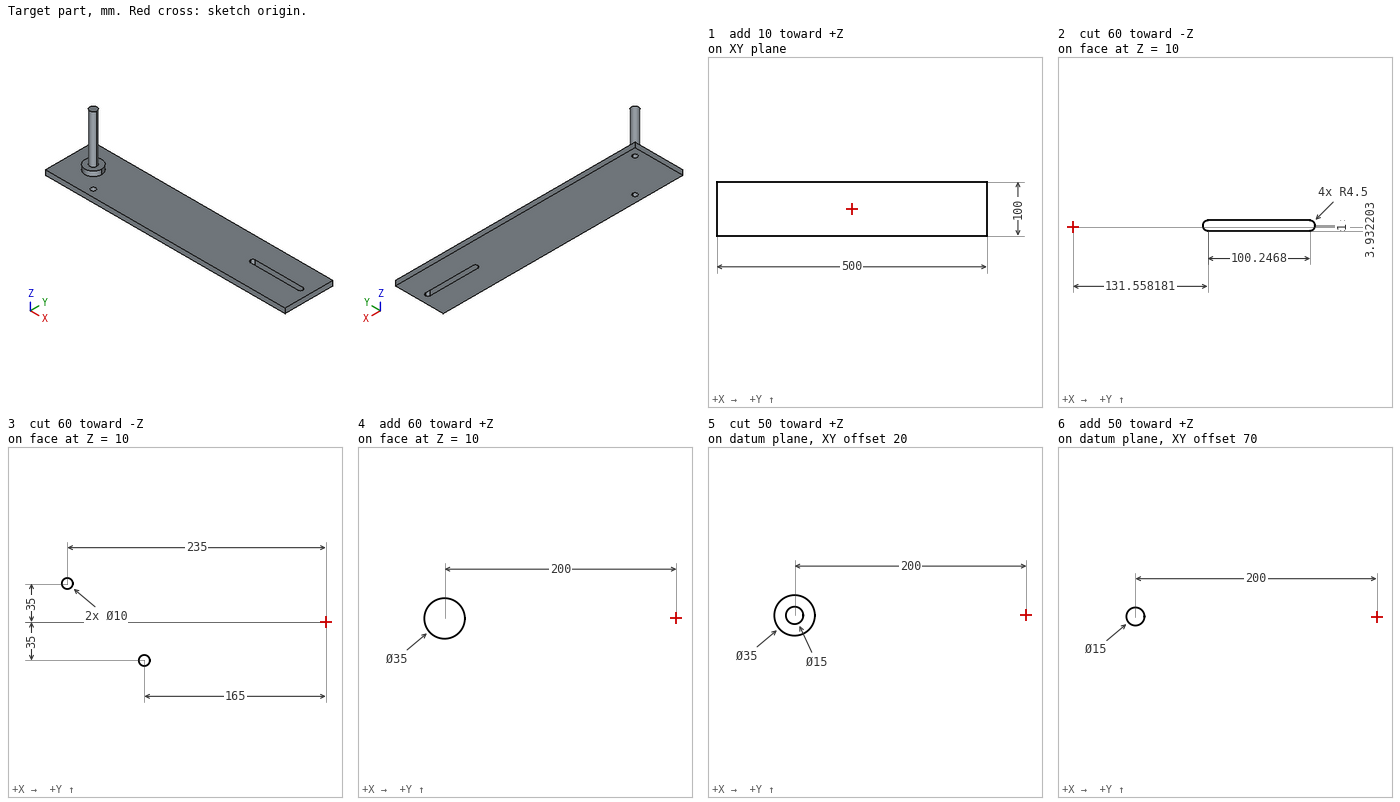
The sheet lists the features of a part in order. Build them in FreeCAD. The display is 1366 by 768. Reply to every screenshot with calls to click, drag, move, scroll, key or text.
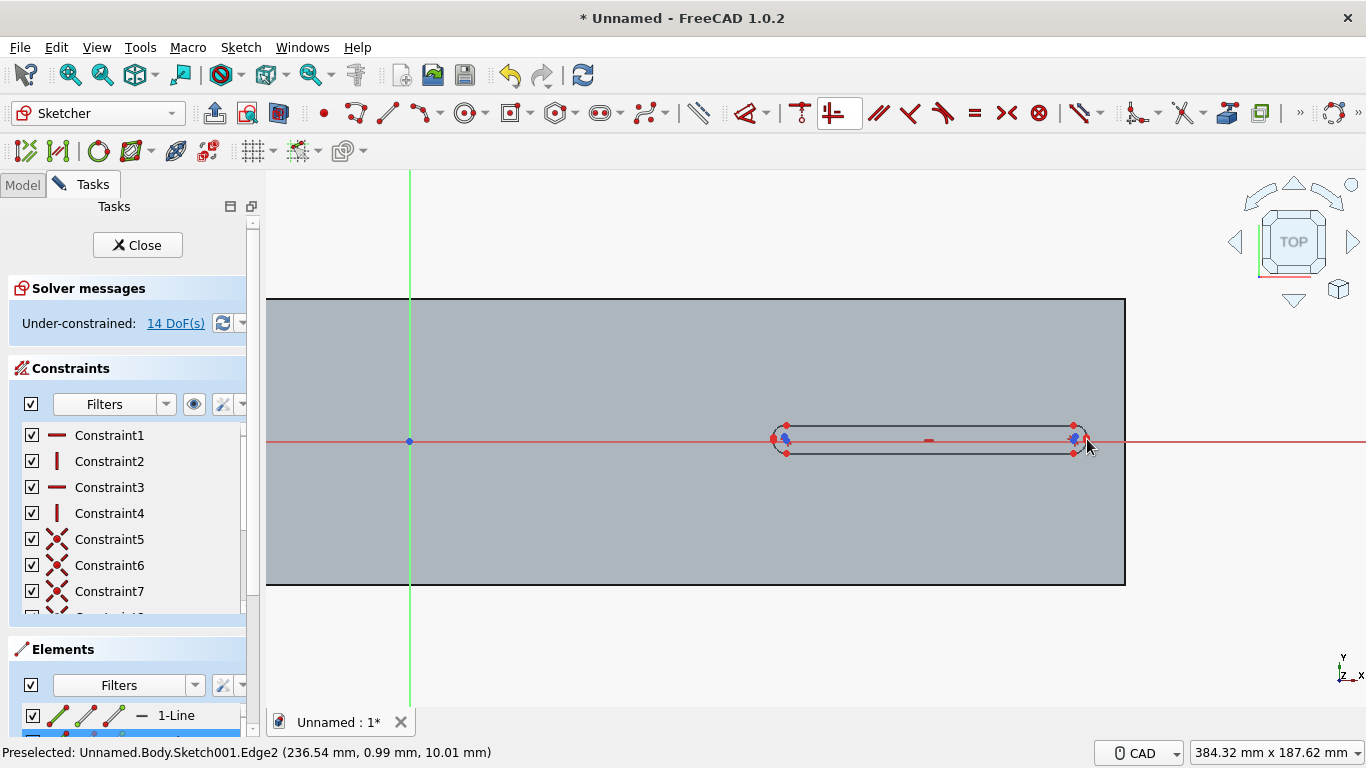
scroll(1079, 452, up, 5)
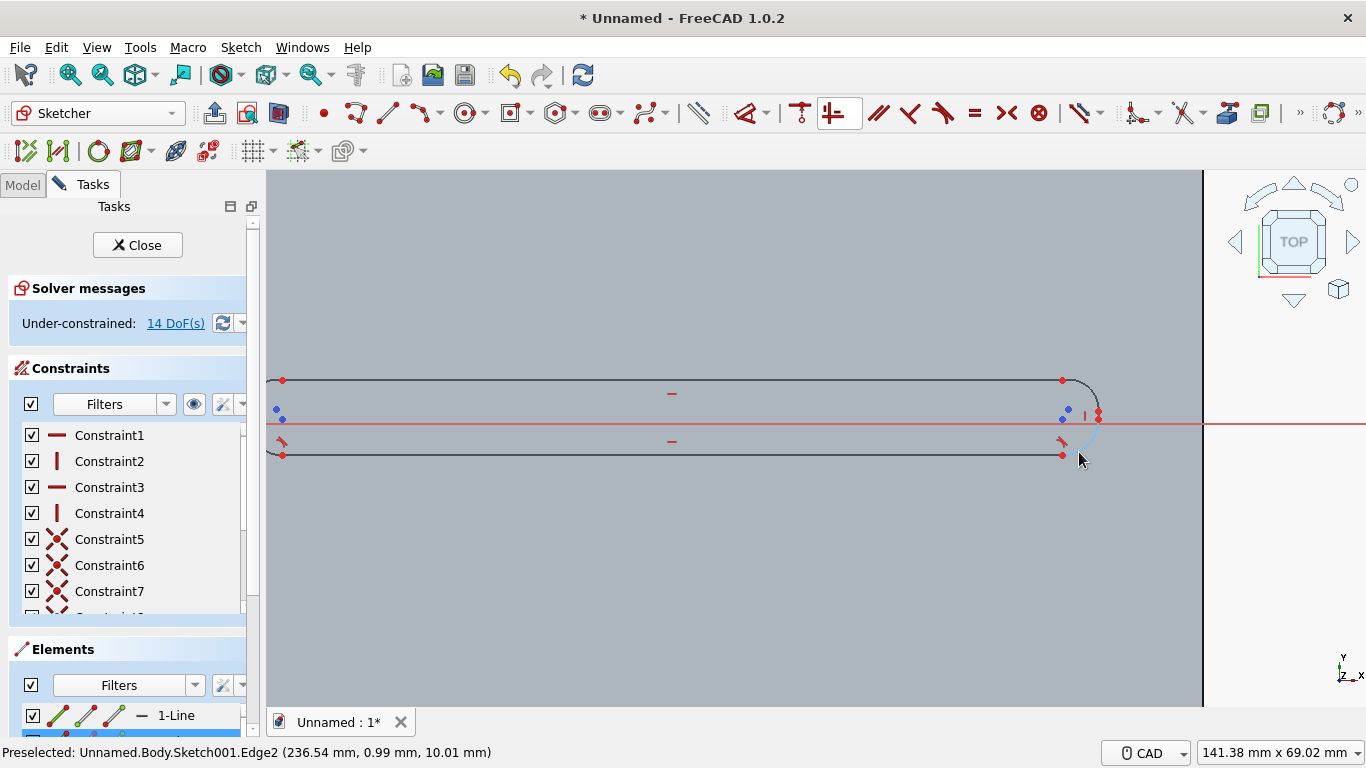
click(1079, 451)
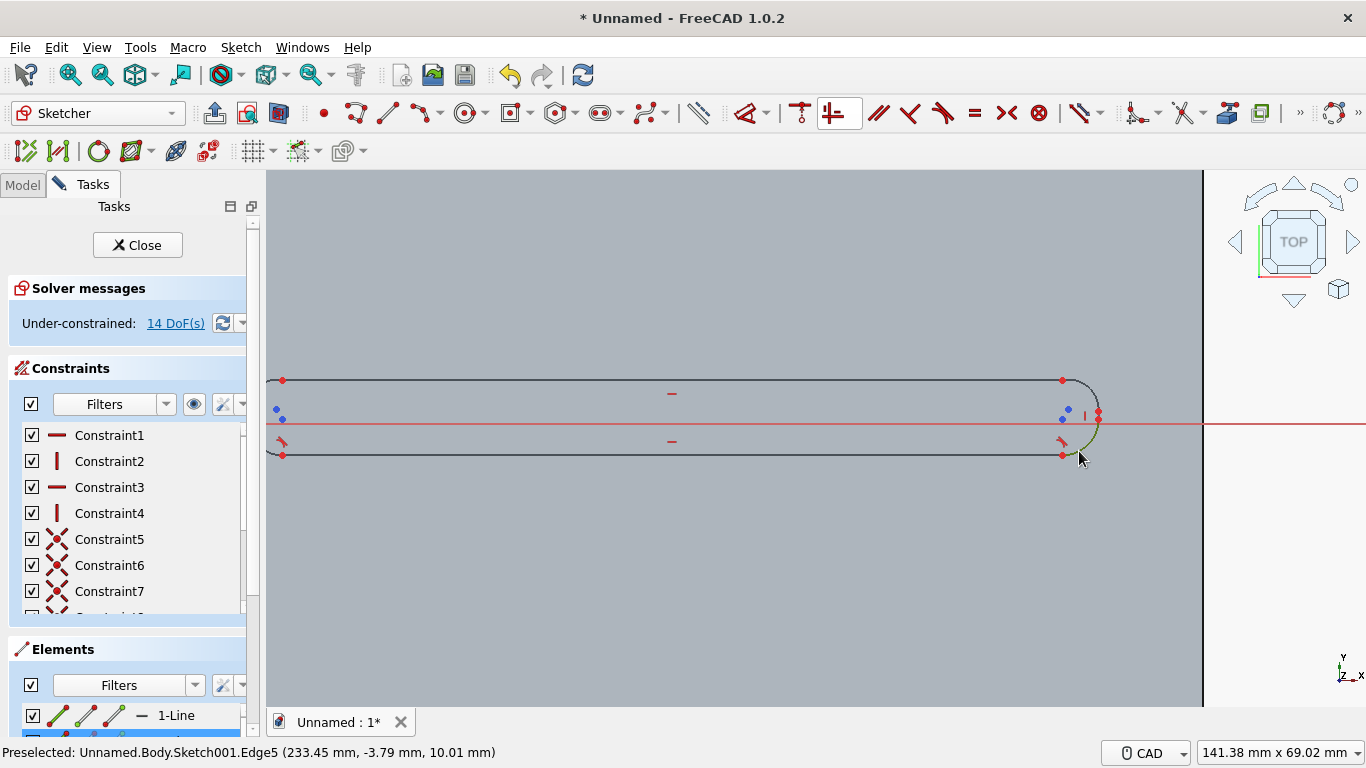
key(t)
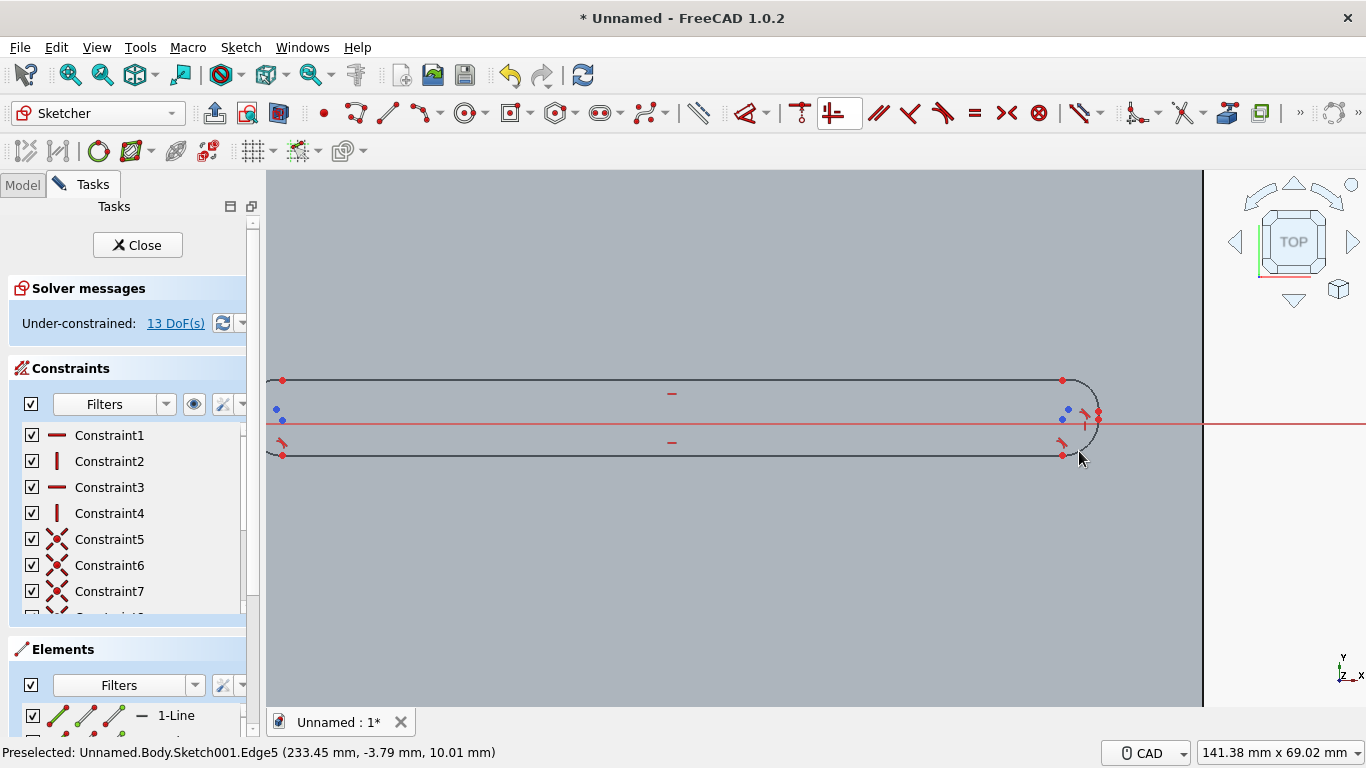
scroll(1099, 416, up, 7)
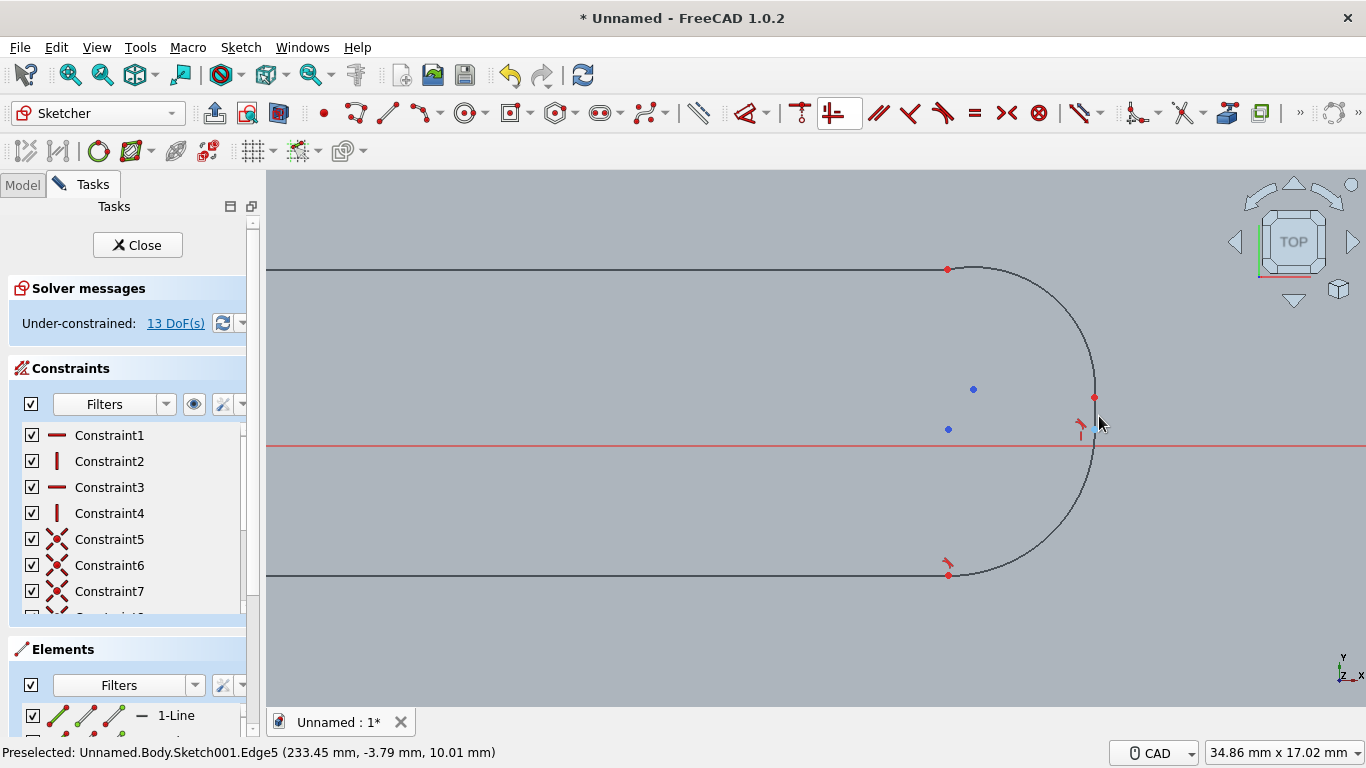
click(1095, 413)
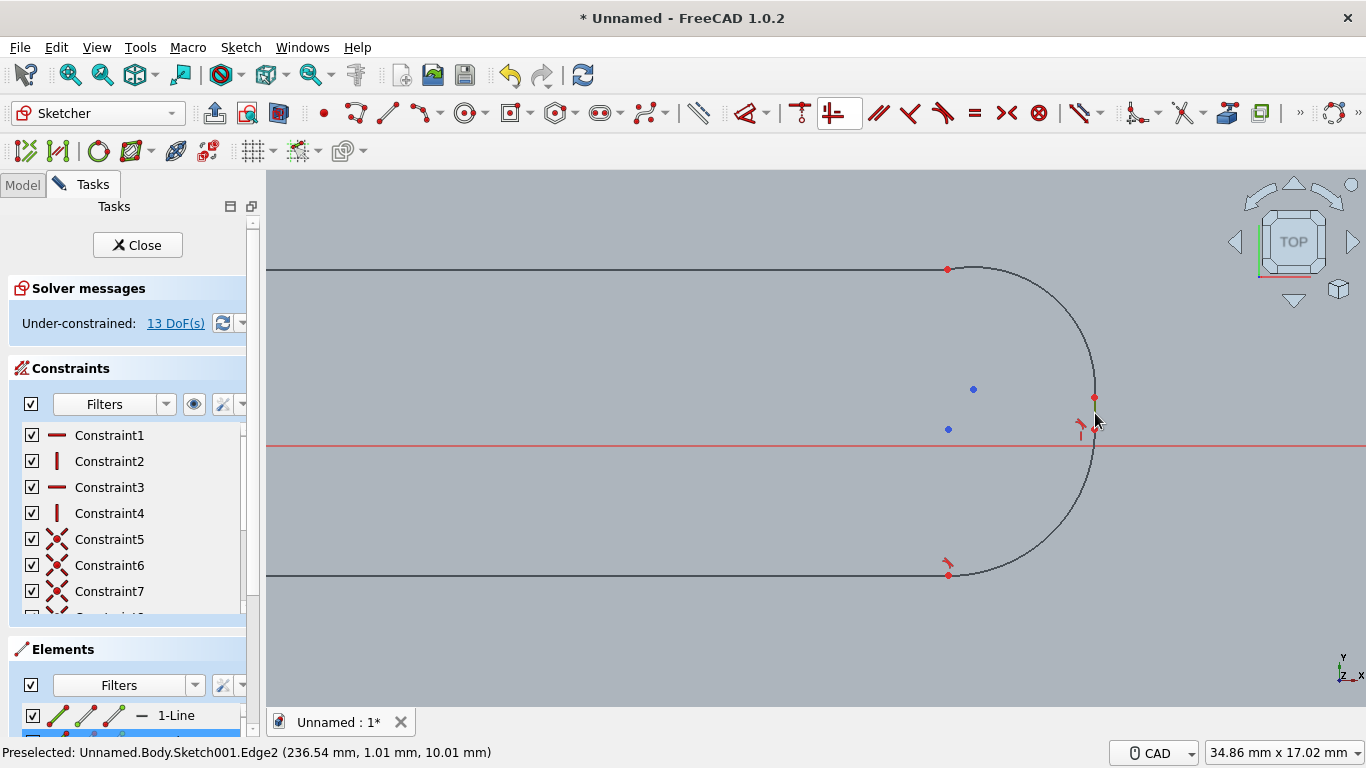
scroll(1085, 441, down, 12)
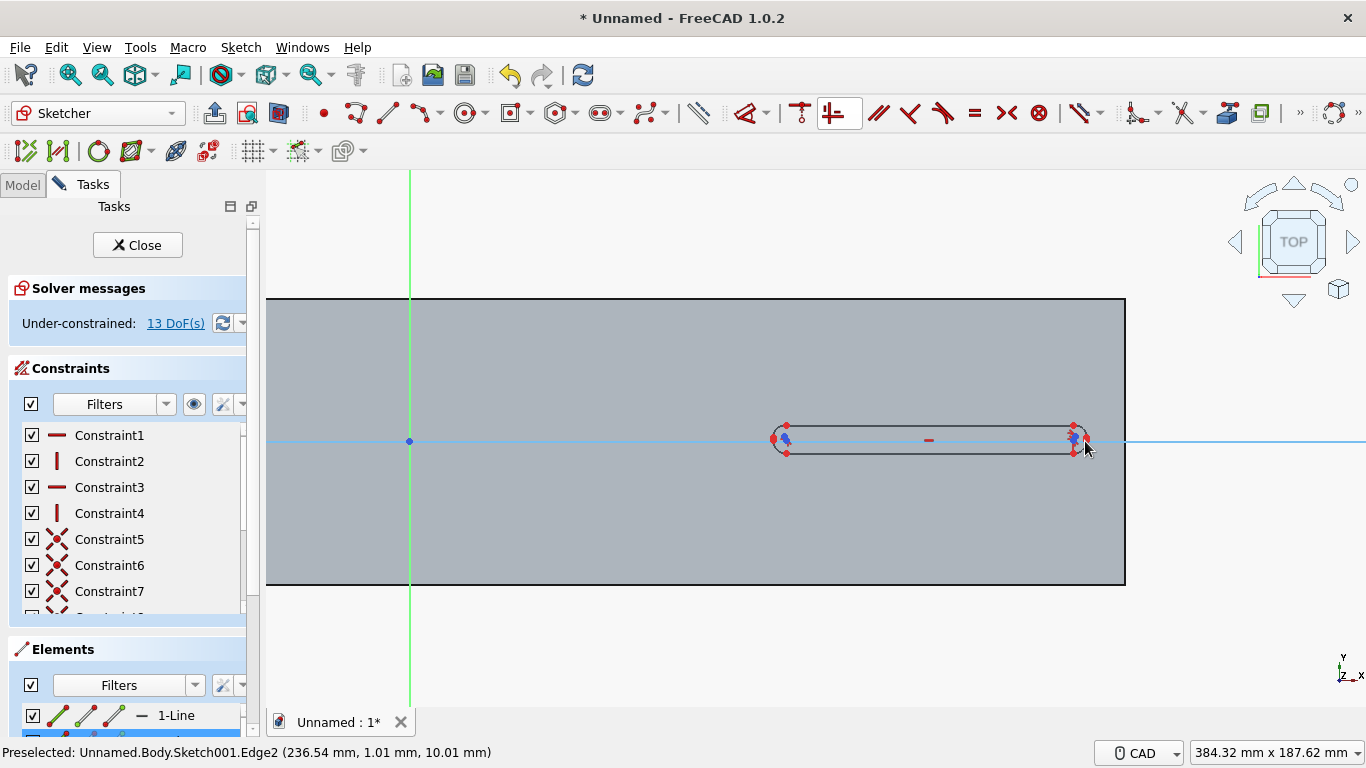
scroll(1085, 432, up, 5)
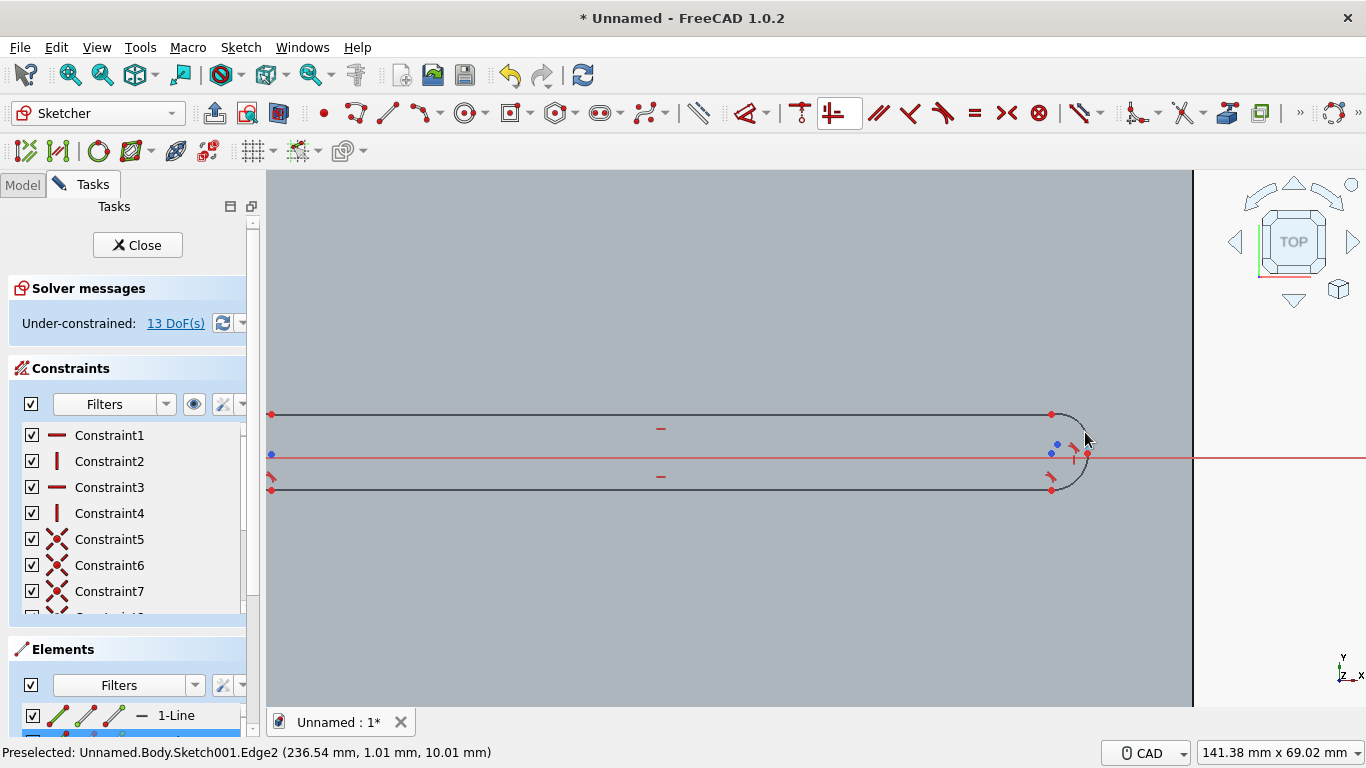
click(1085, 430)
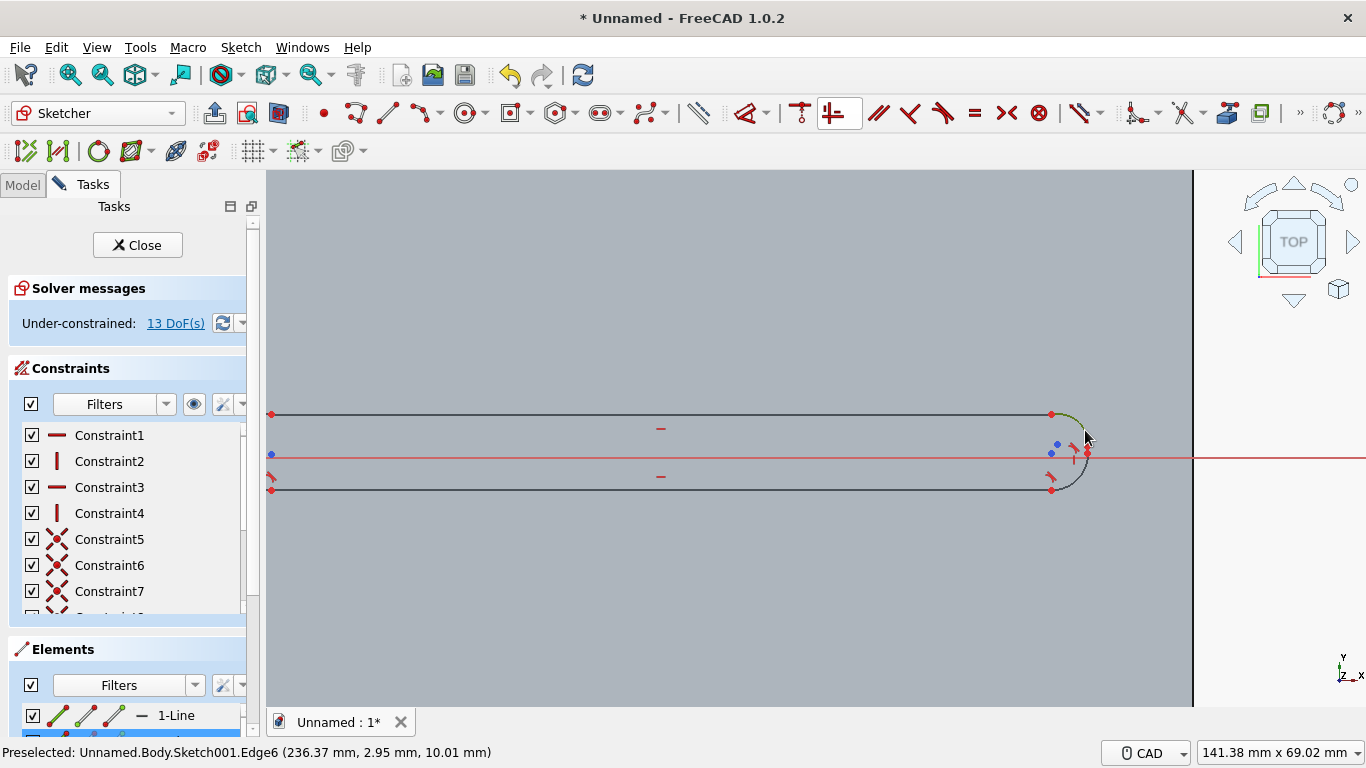
key(t)